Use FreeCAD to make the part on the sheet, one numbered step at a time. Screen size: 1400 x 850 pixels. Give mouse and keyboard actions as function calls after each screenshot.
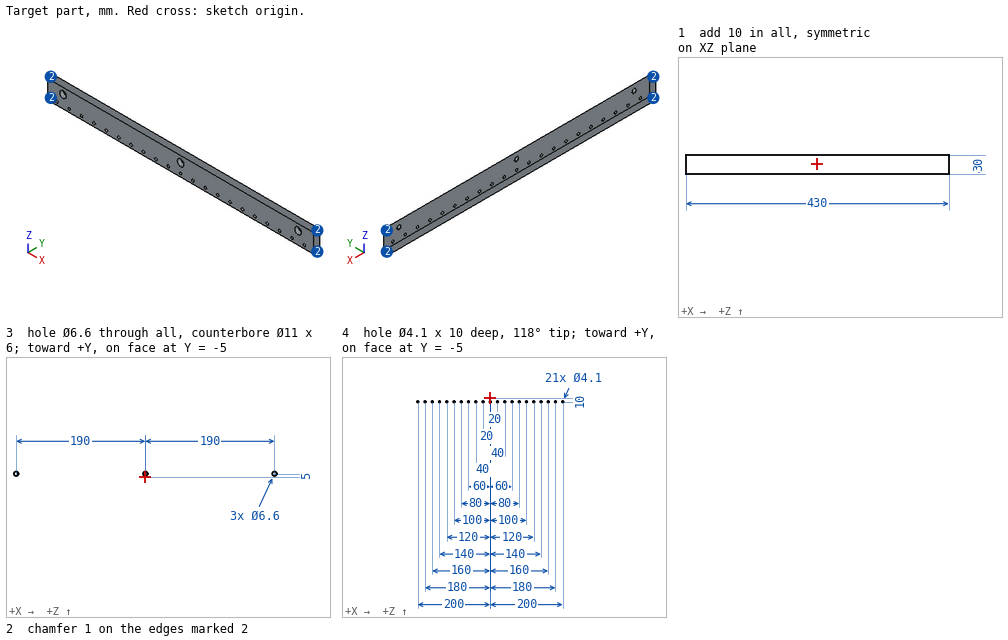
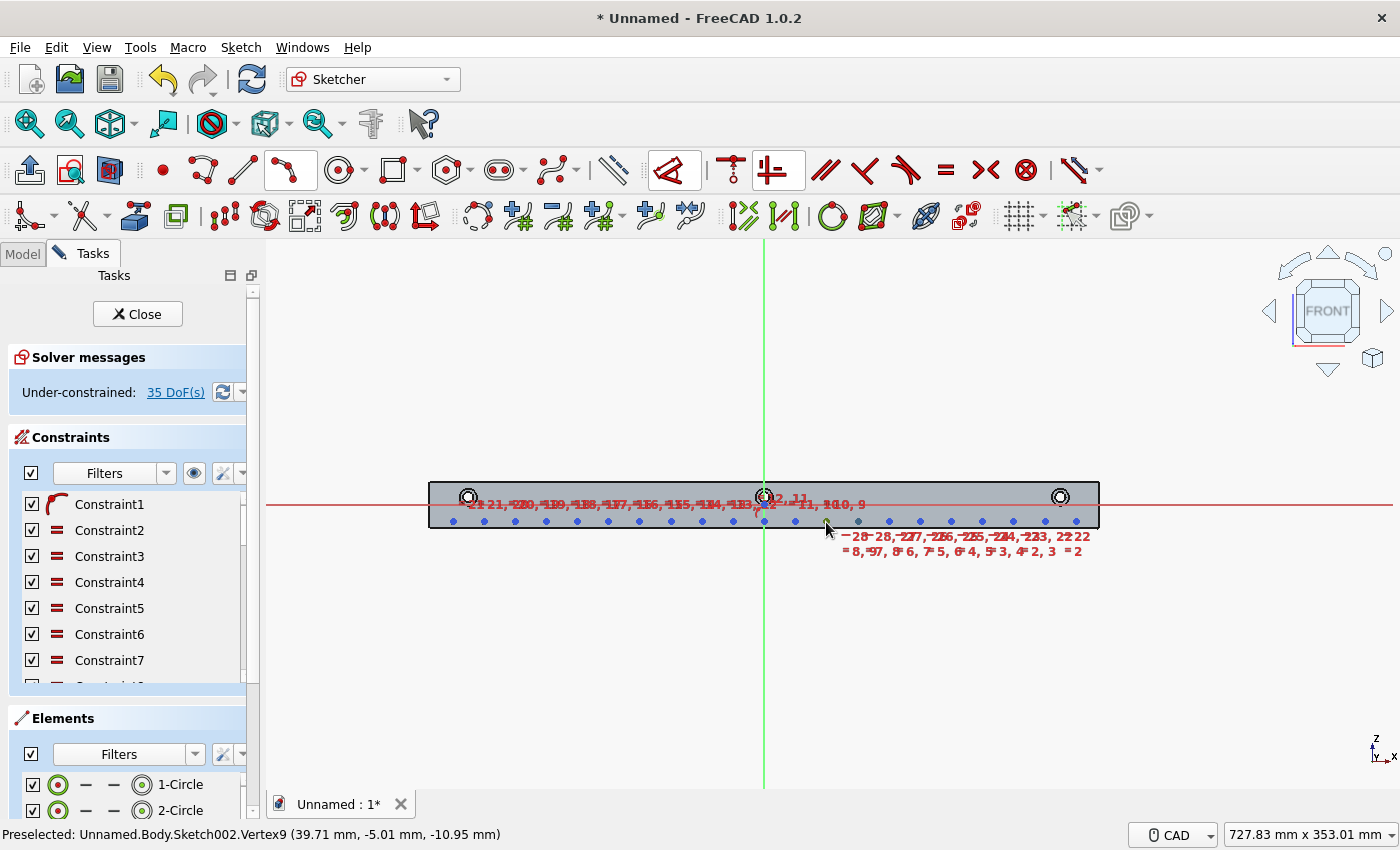
click(800, 170)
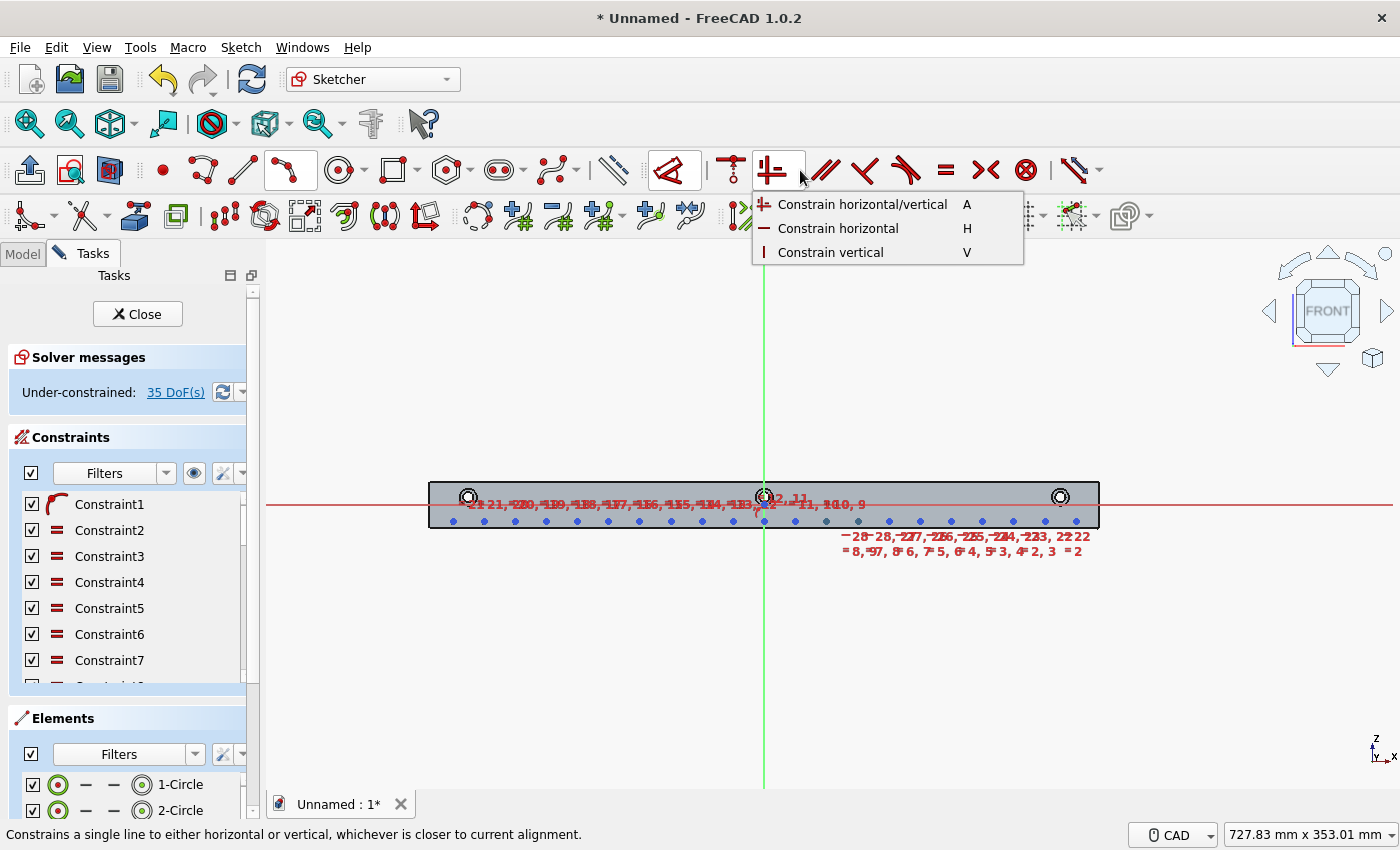
click(888, 228)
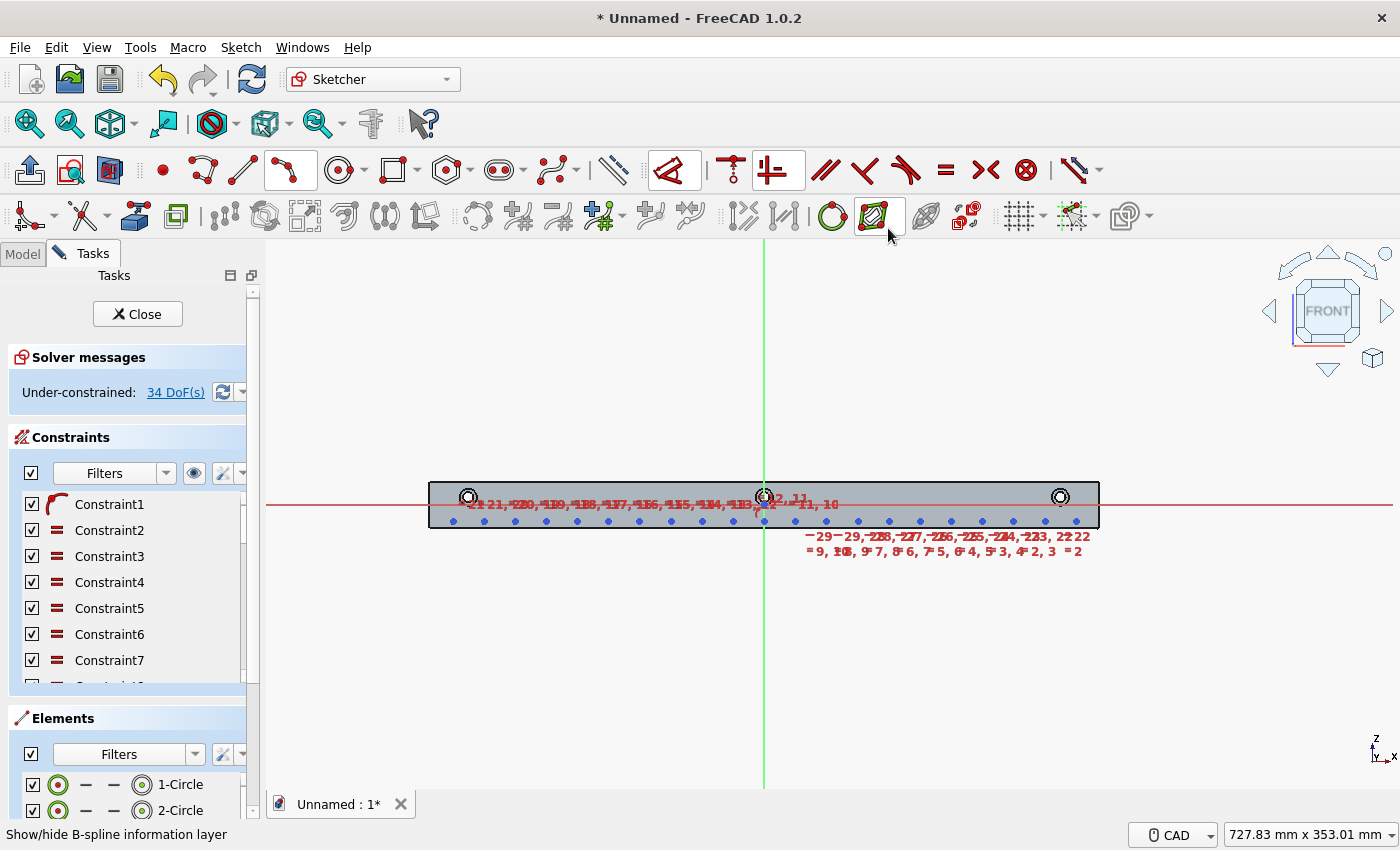
click(826, 522)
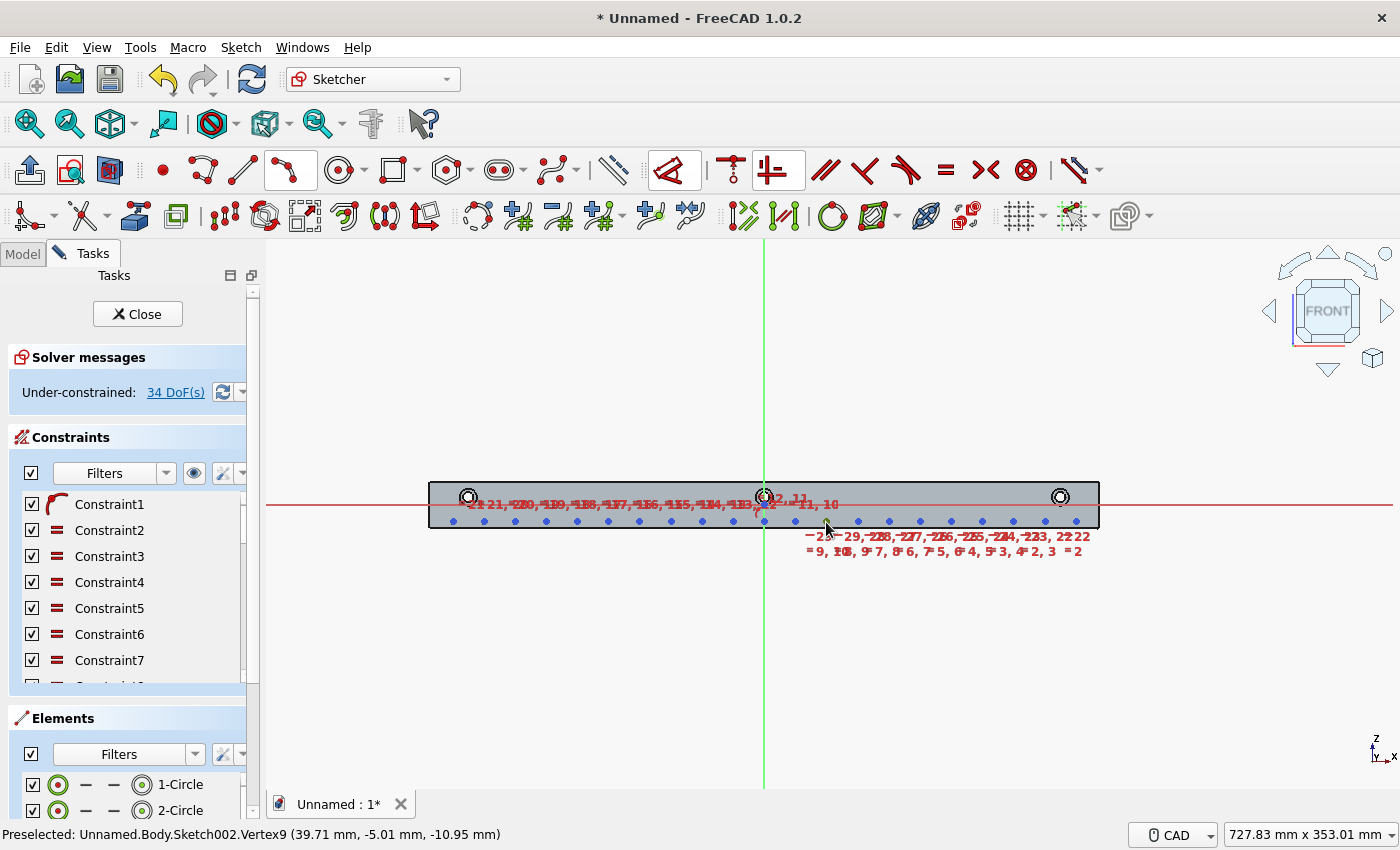
click(795, 522)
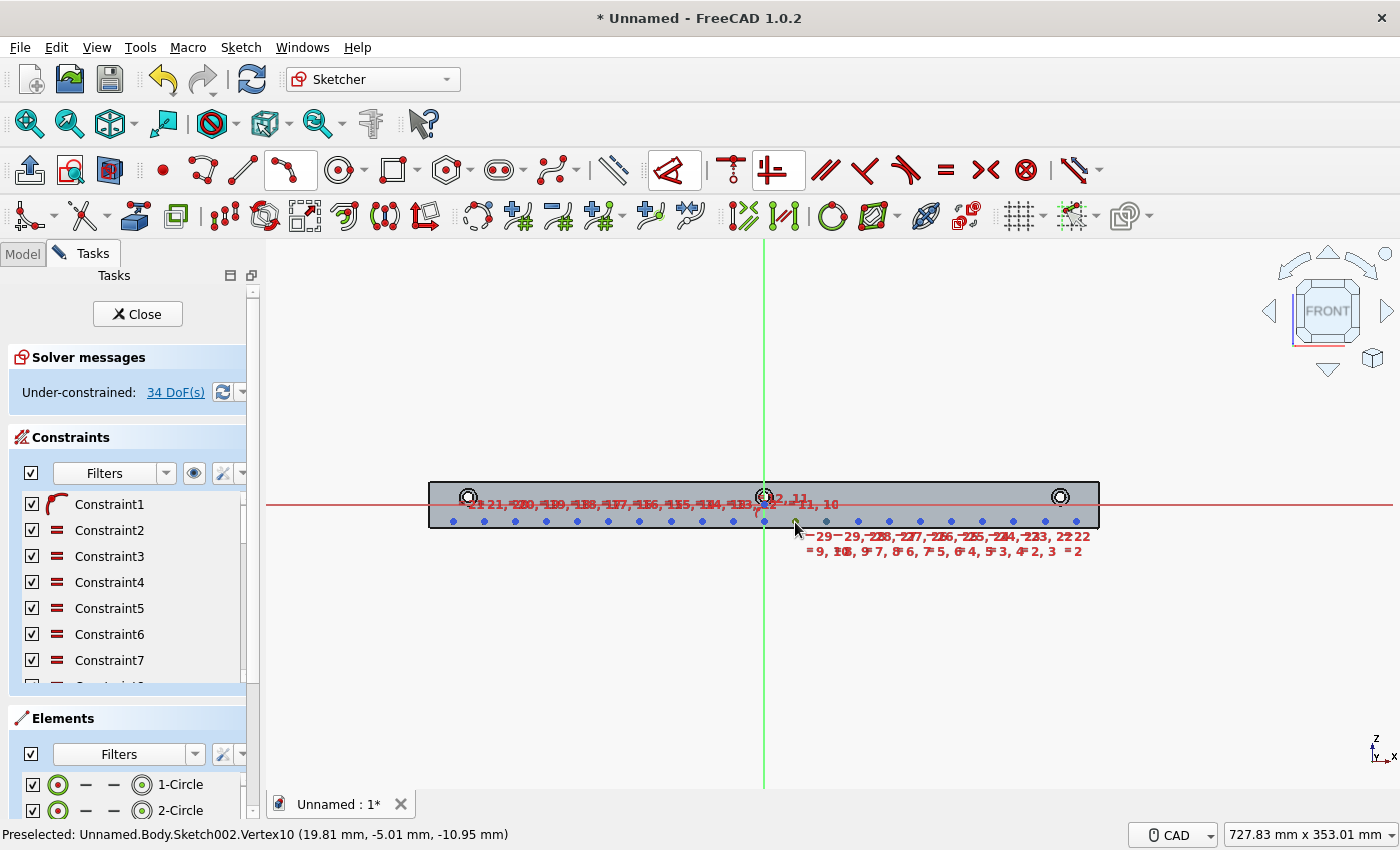
click(800, 170)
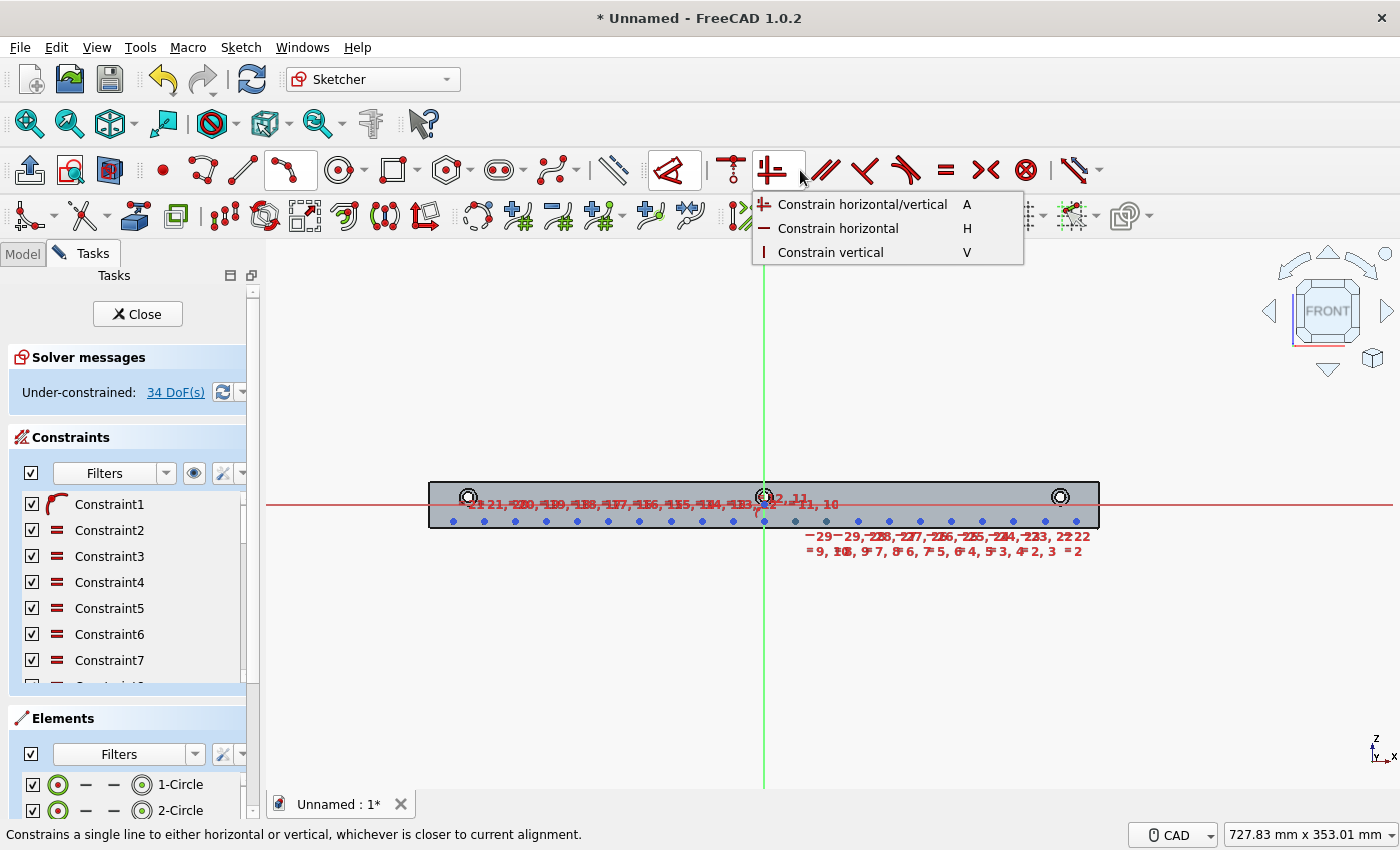
click(888, 228)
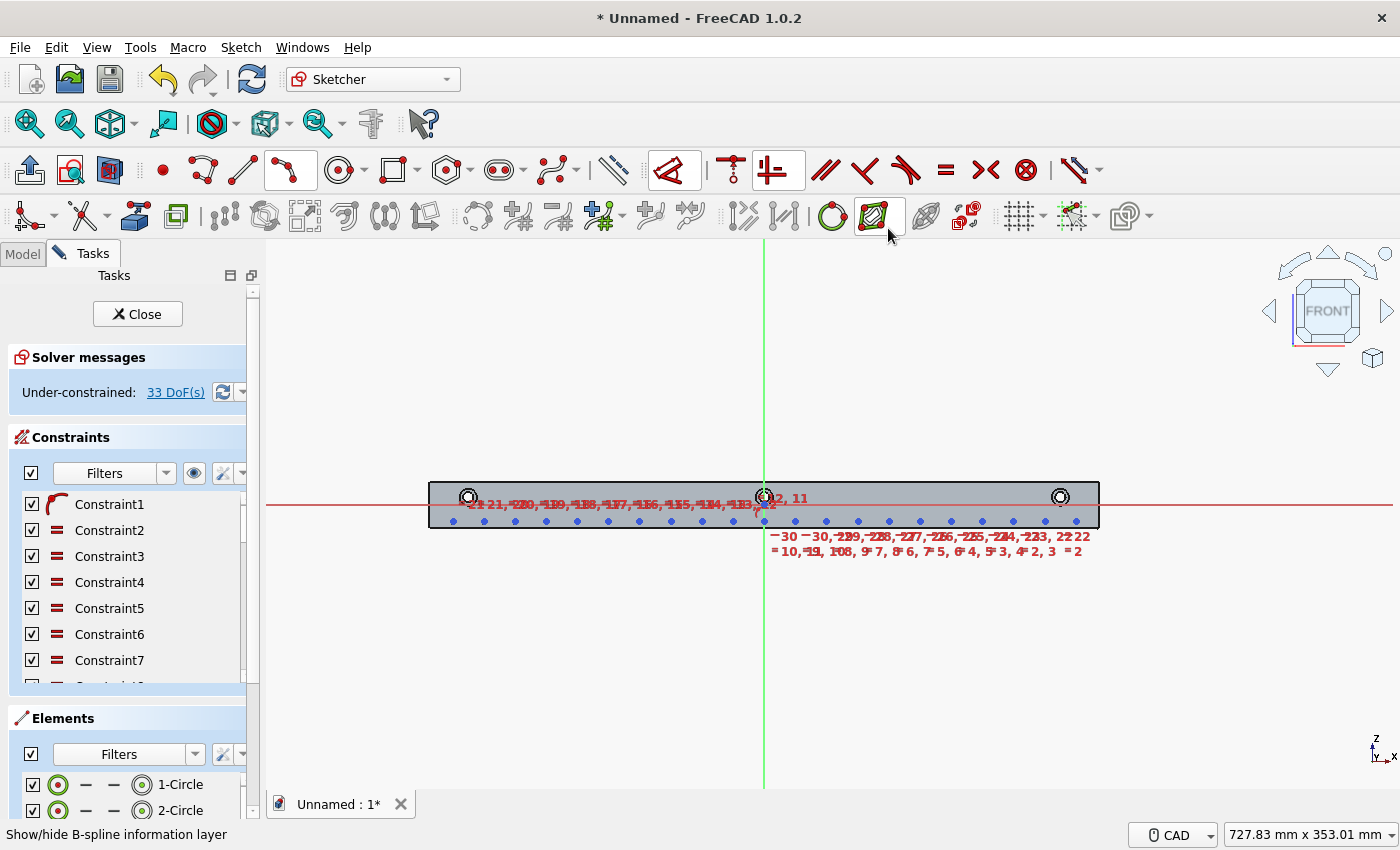
click(795, 522)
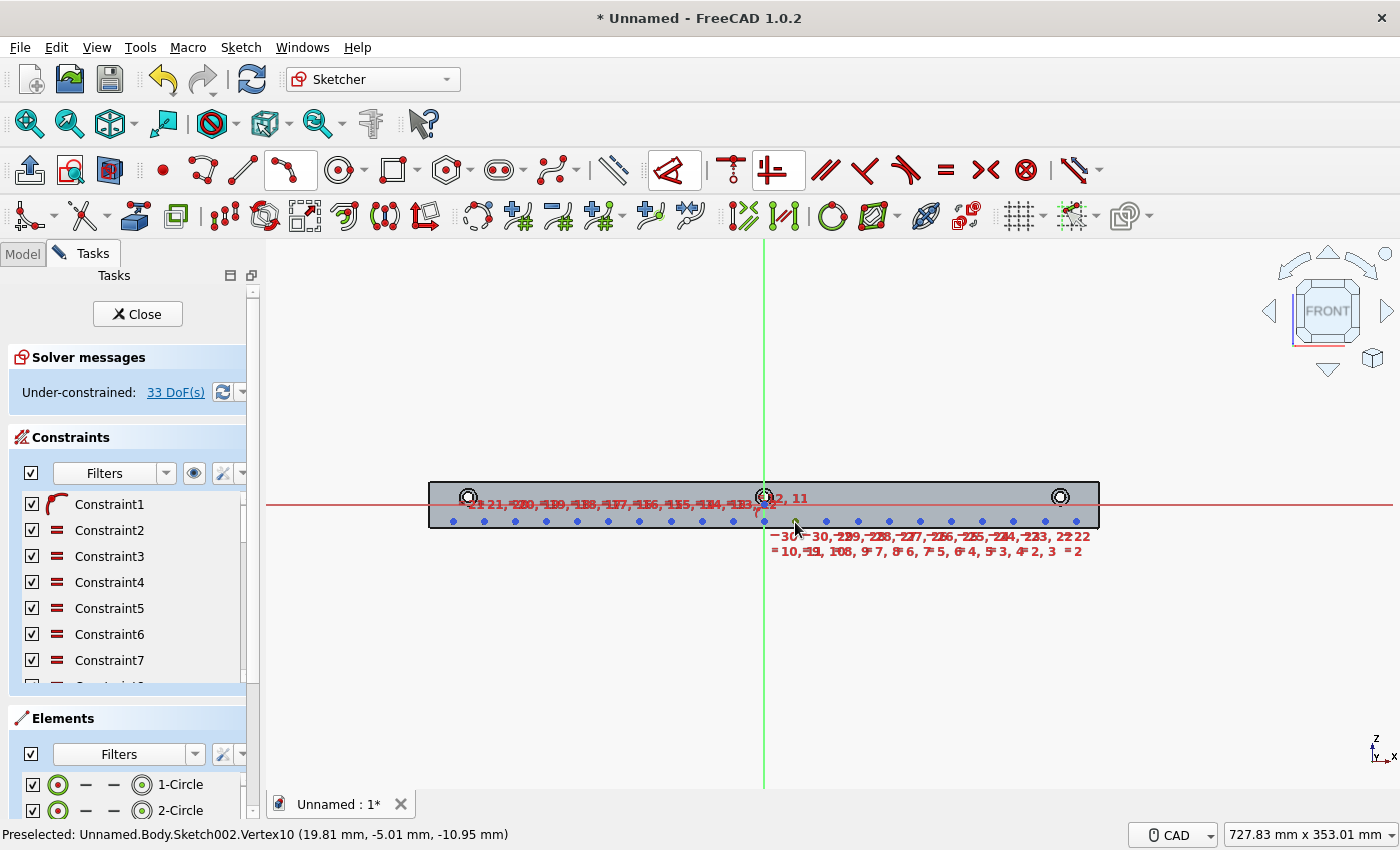
click(764, 522)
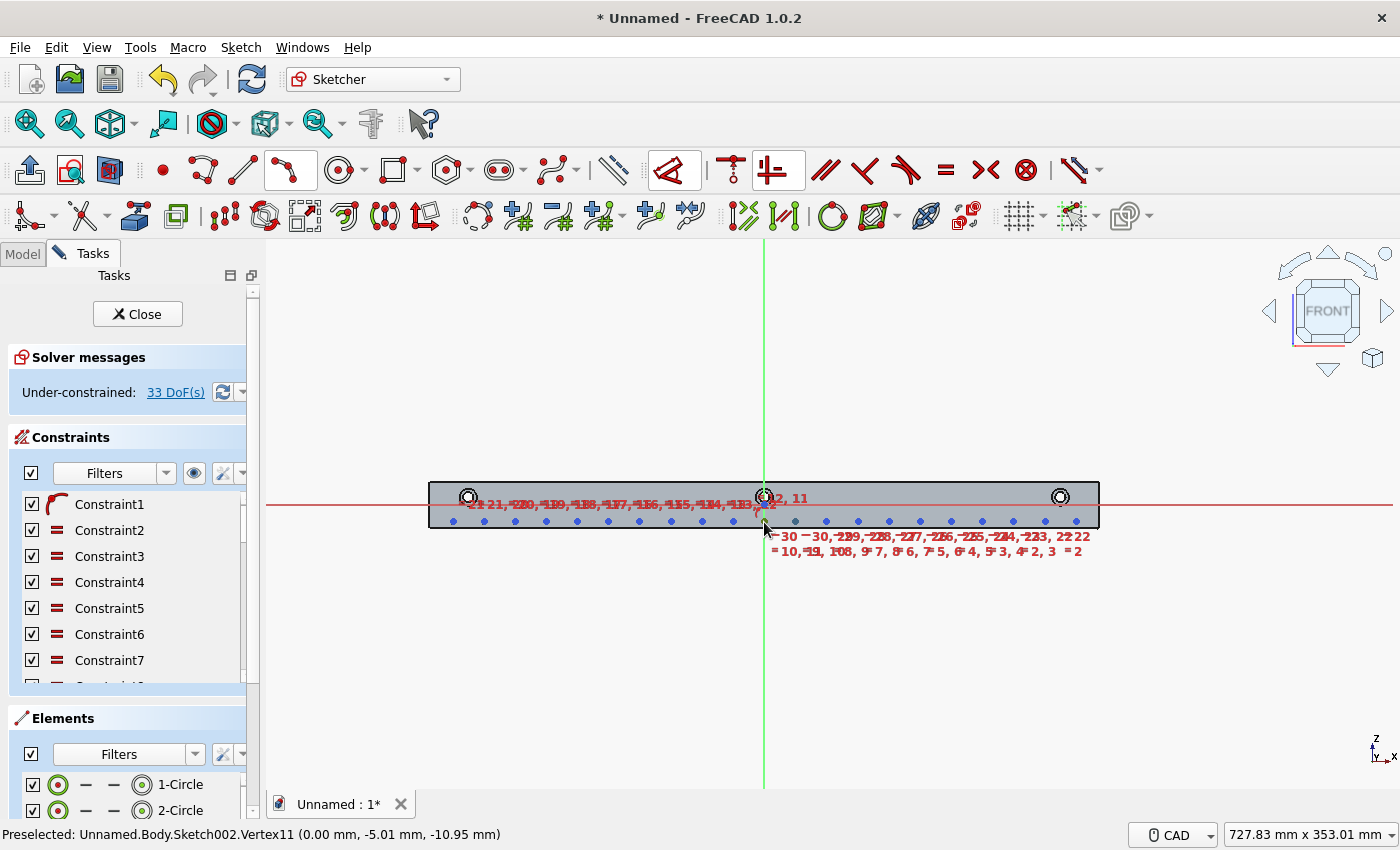
click(800, 170)